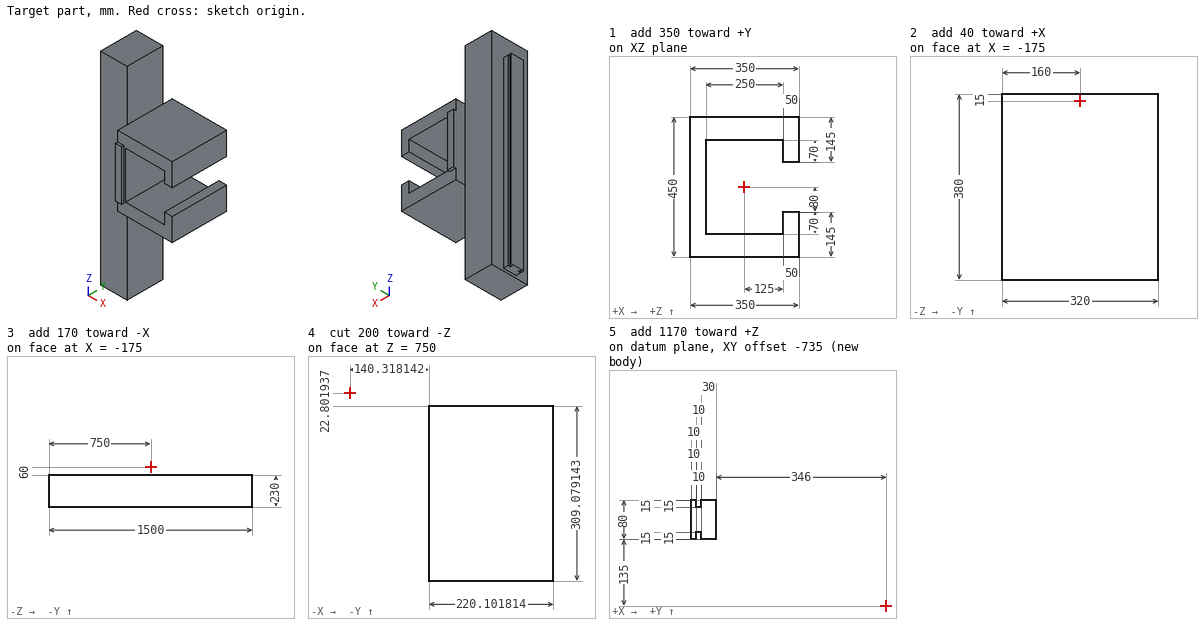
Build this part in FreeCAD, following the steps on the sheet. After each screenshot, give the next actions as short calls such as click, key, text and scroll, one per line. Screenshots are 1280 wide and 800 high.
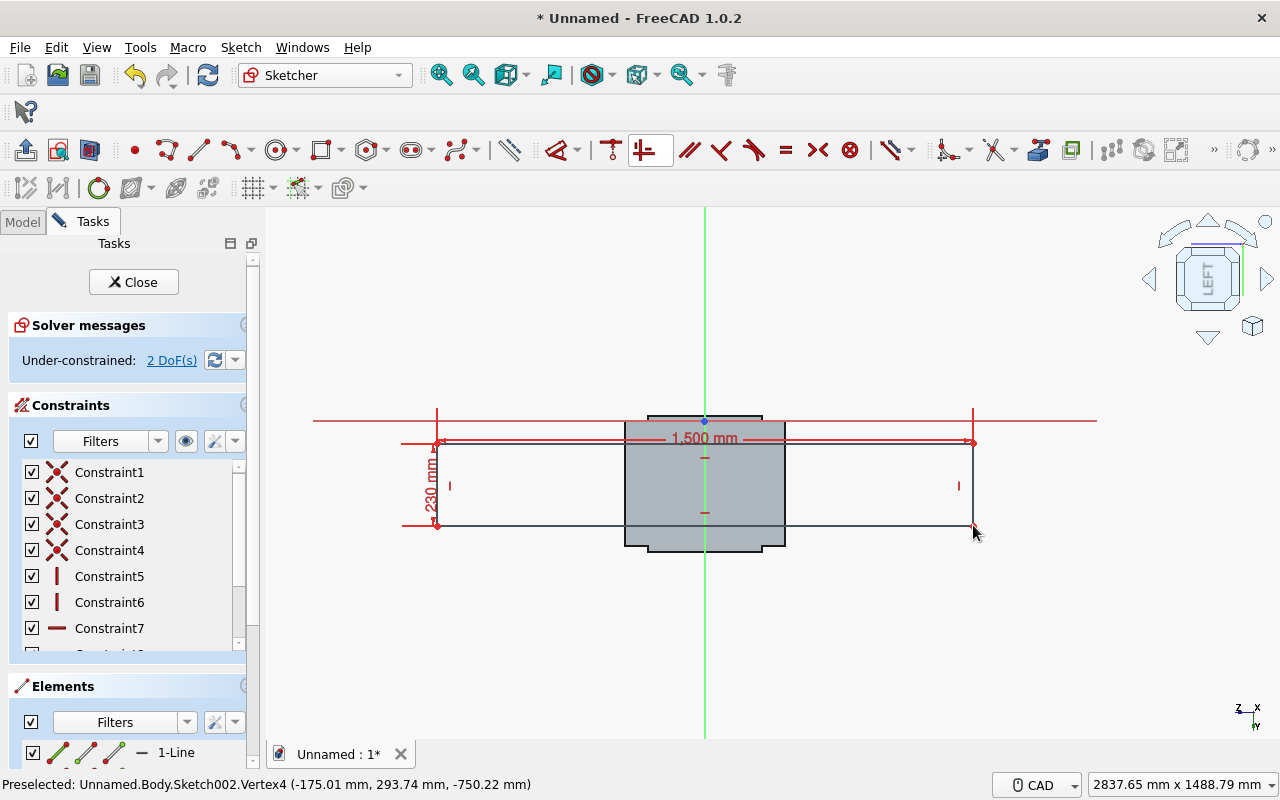
click(556, 150)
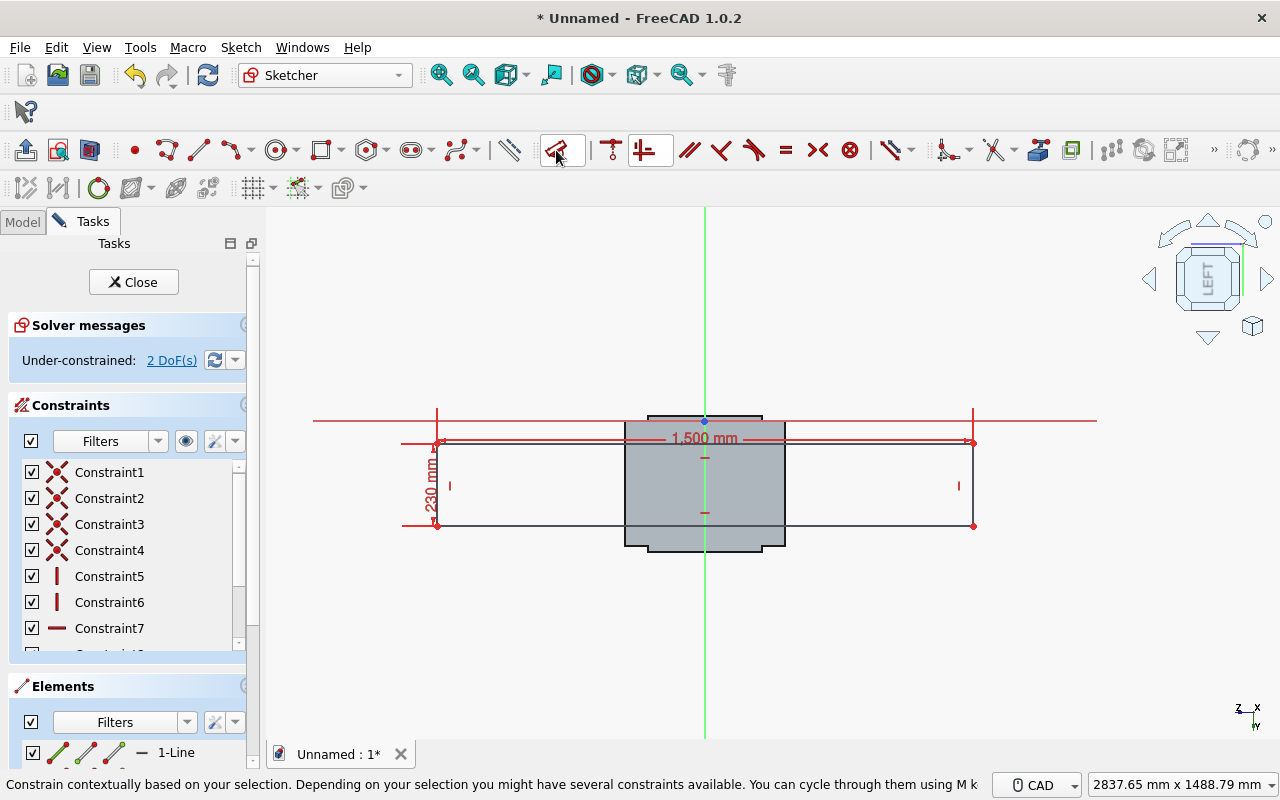
scroll(437, 444, up, 4)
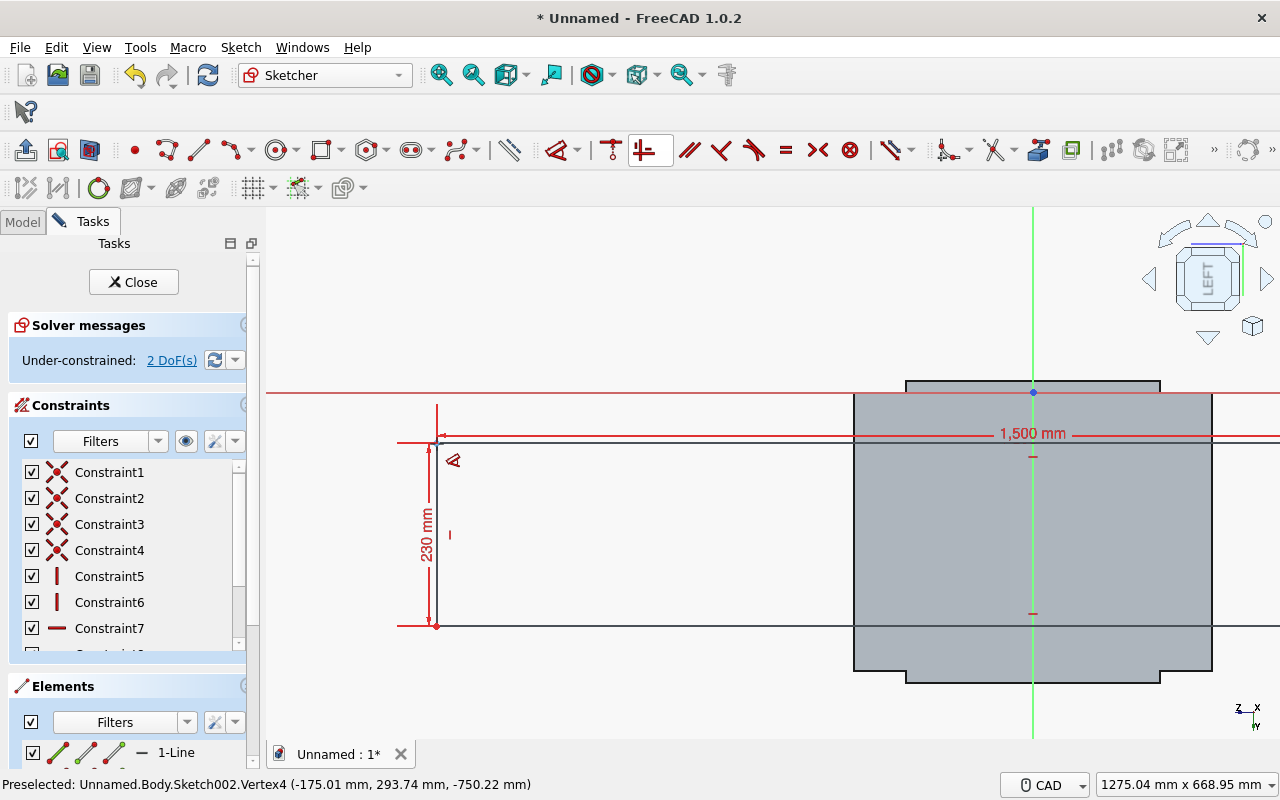
click(437, 443)
click(403, 418)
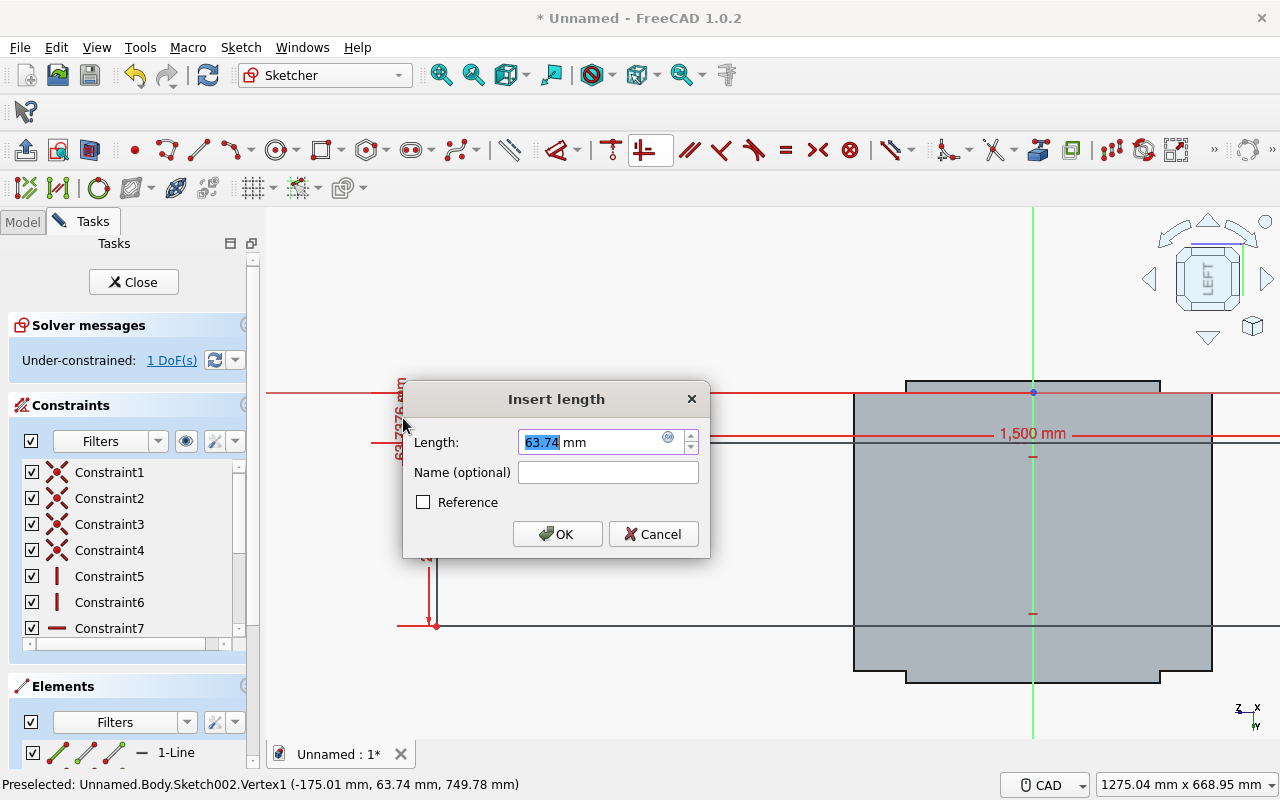
text(60)
key(Return)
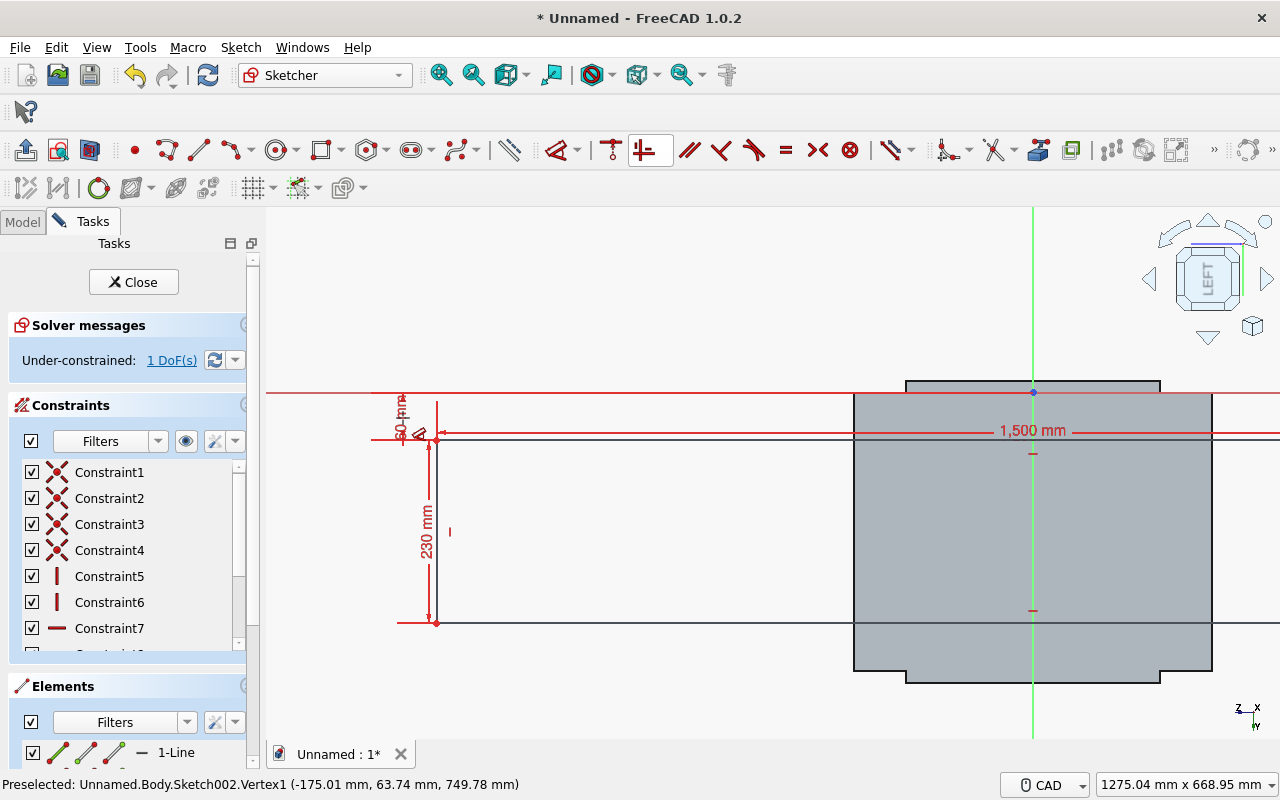
click(437, 440)
click(735, 359)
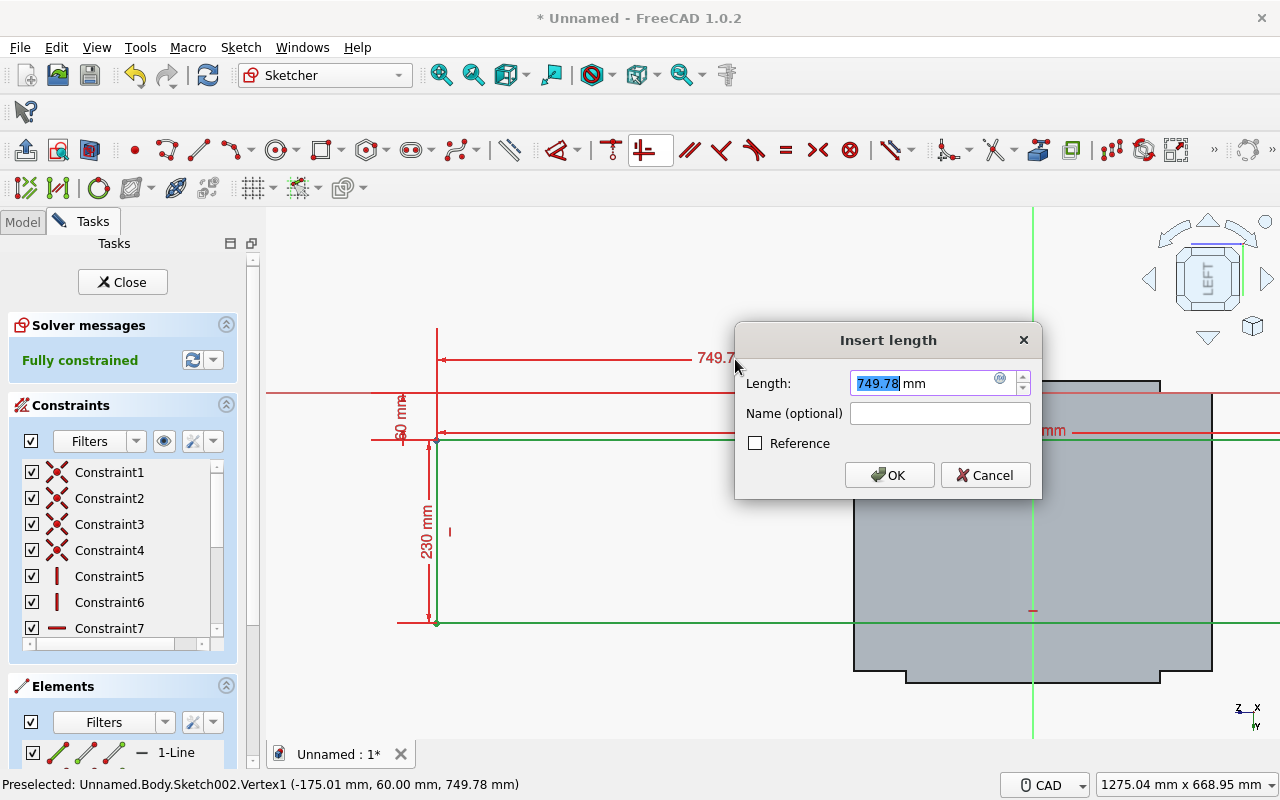
text(750)
key(Return)
key(Escape)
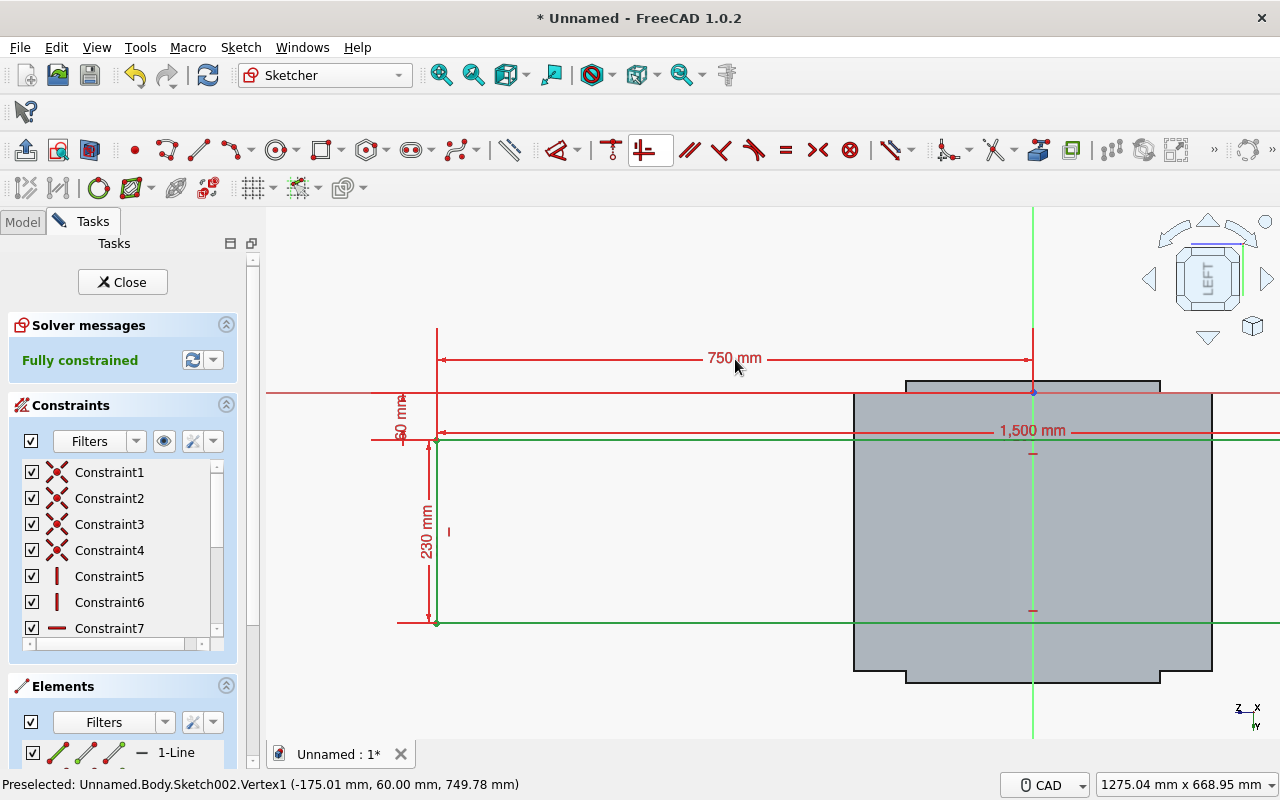
click(123, 282)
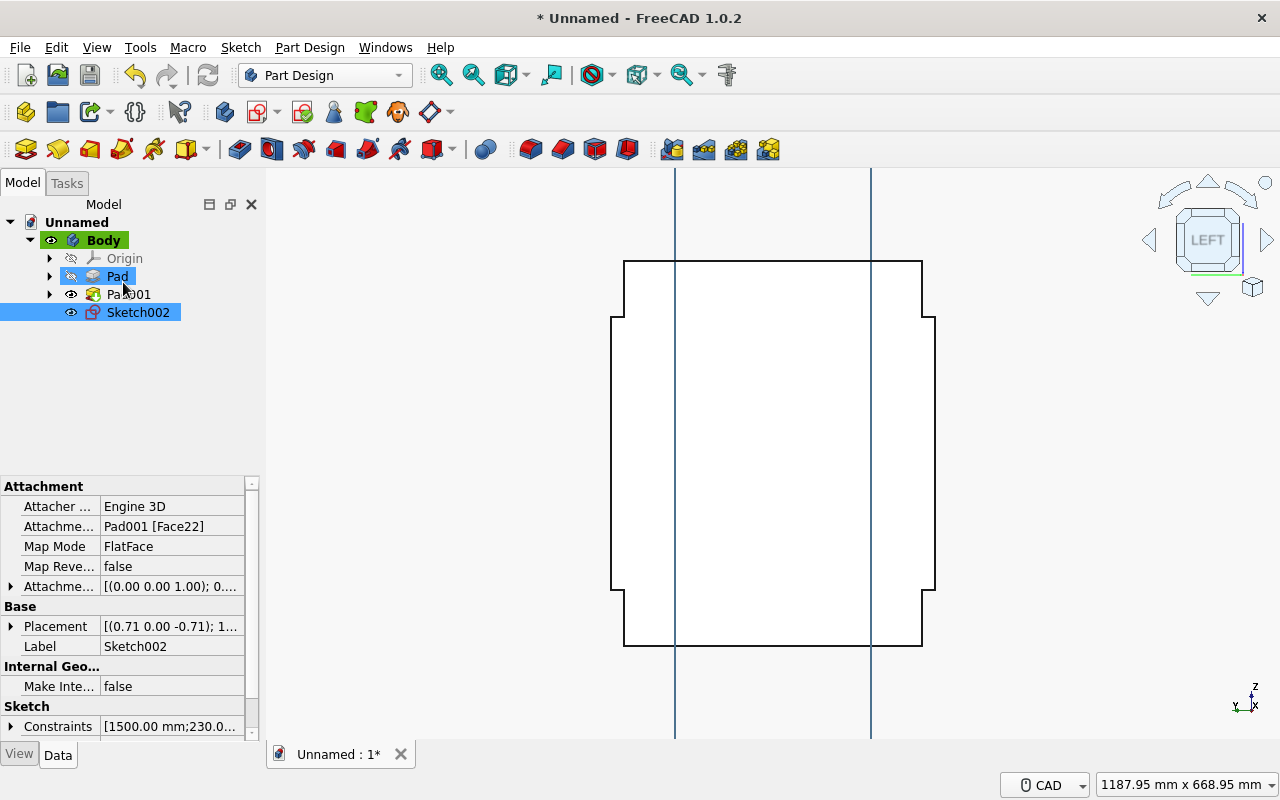
click(26, 150)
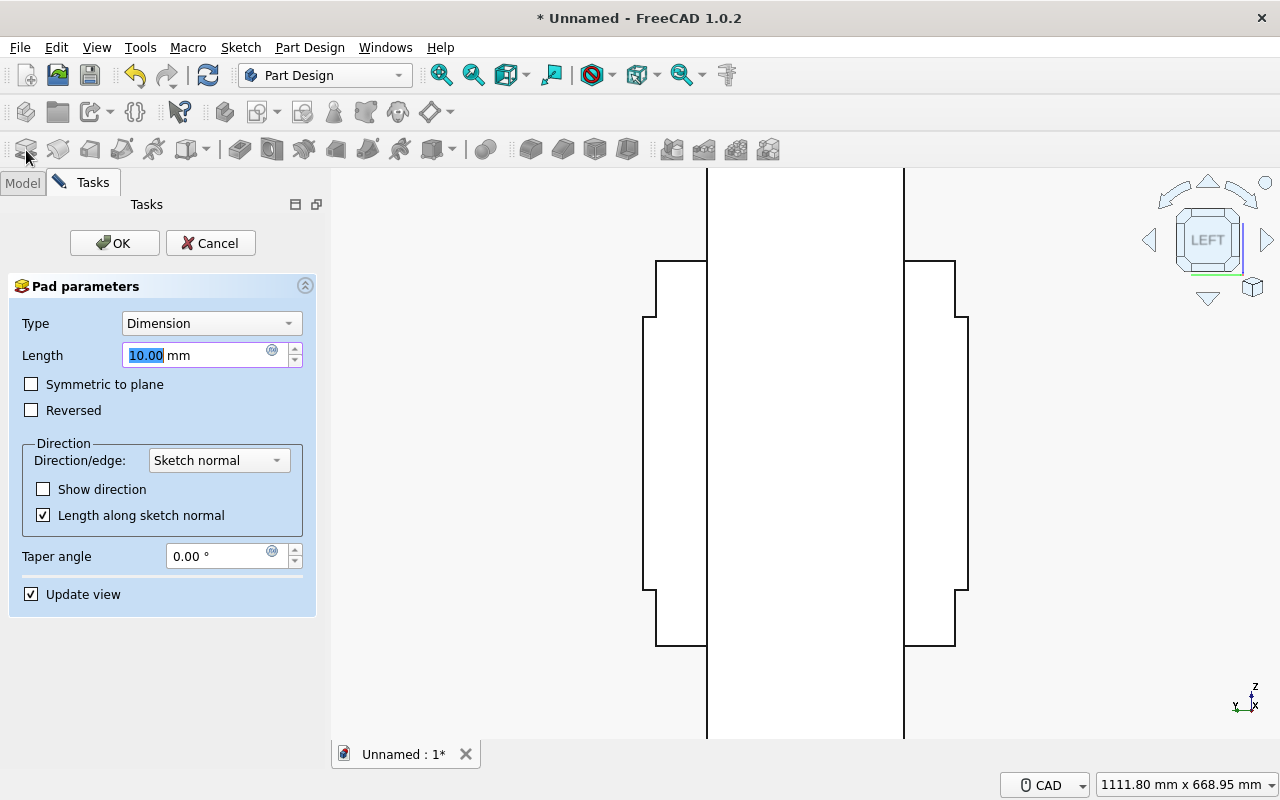
text(170)
key(Tab)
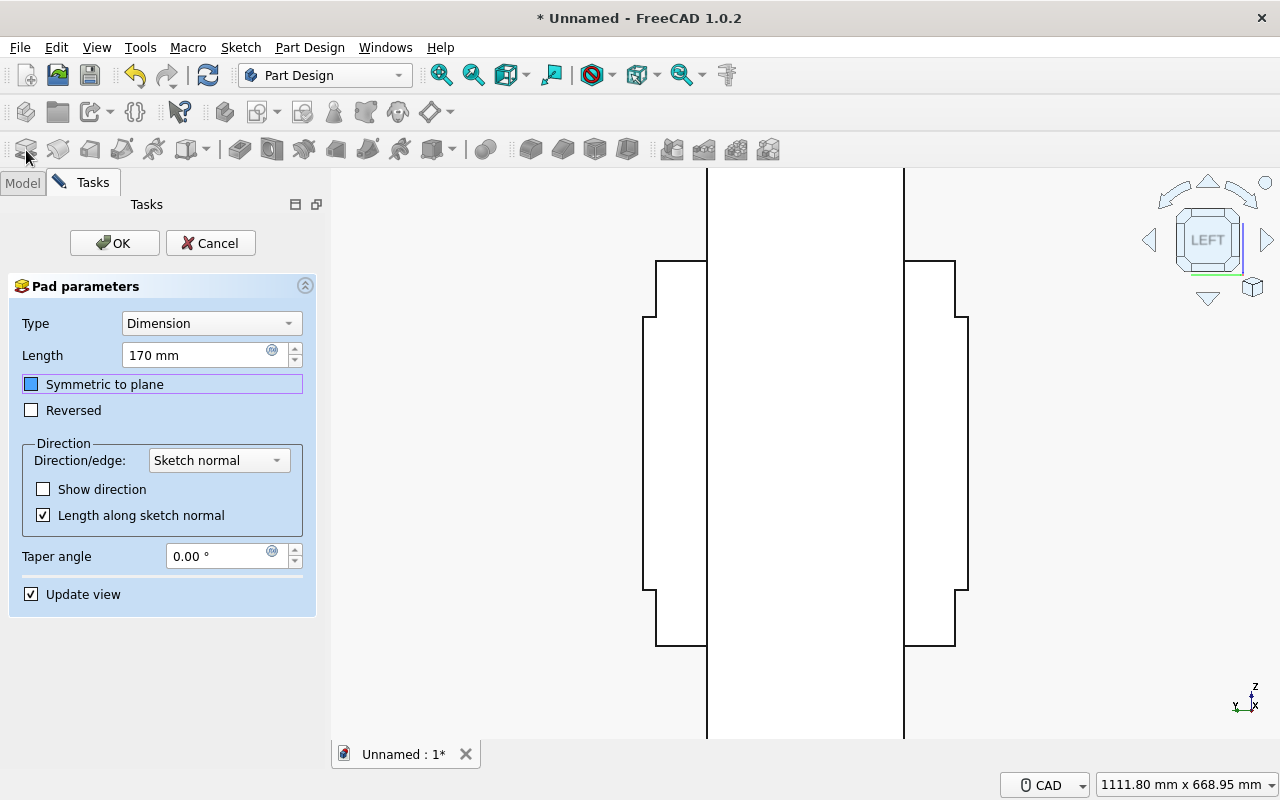
click(115, 243)